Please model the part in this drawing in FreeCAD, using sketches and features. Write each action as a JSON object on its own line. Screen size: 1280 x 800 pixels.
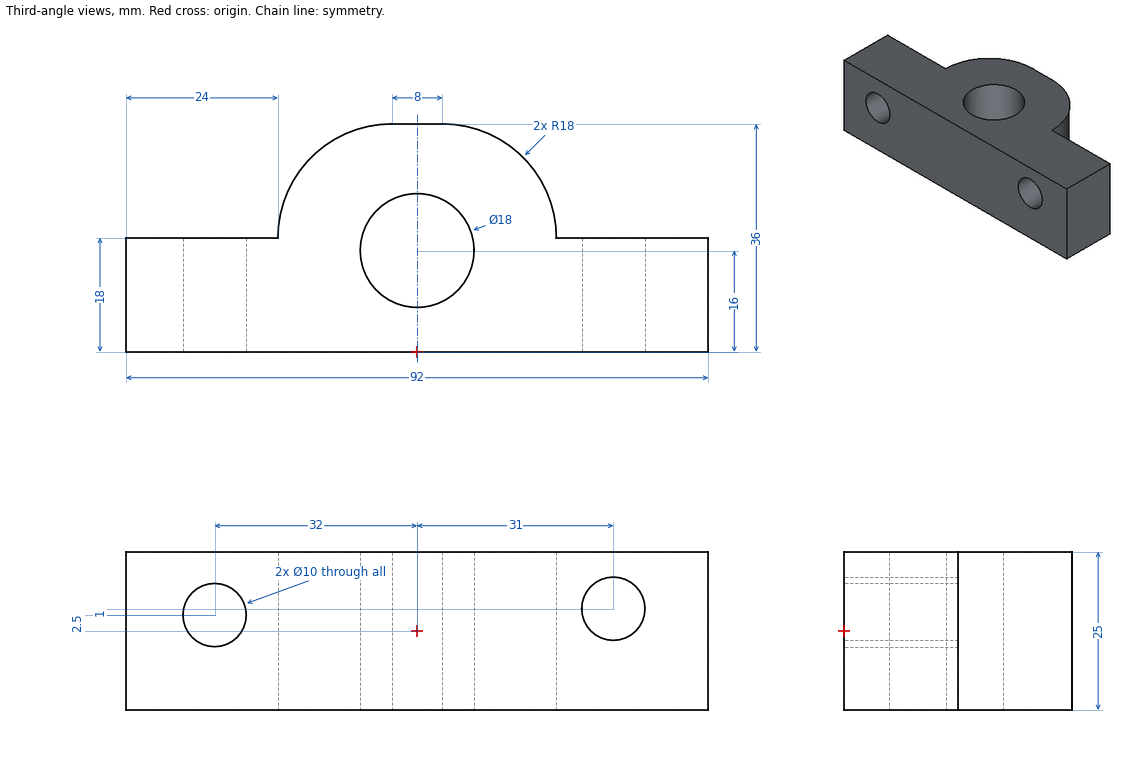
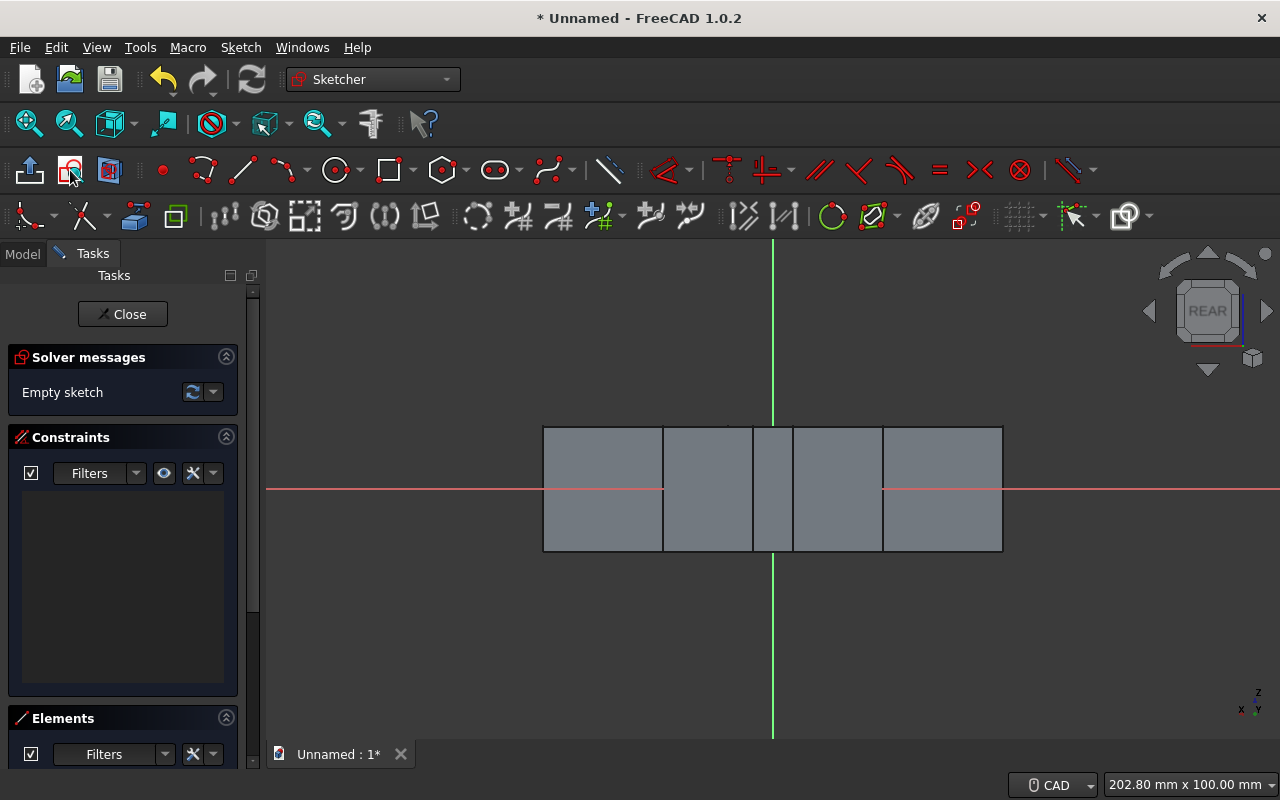
{"action": "key", "text": "q s"}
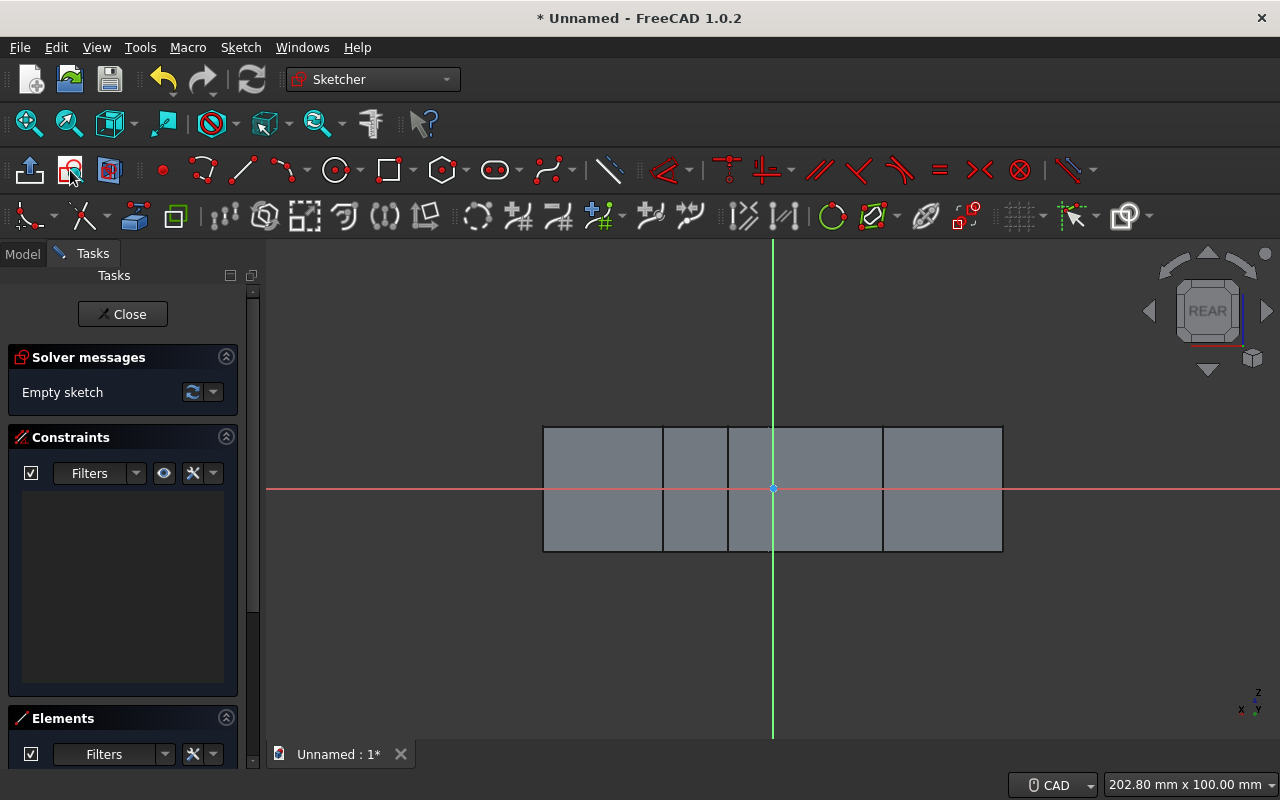
{"action": "scroll", "coordinate": [920, 444], "scroll_direction": "up", "scroll_amount": 2}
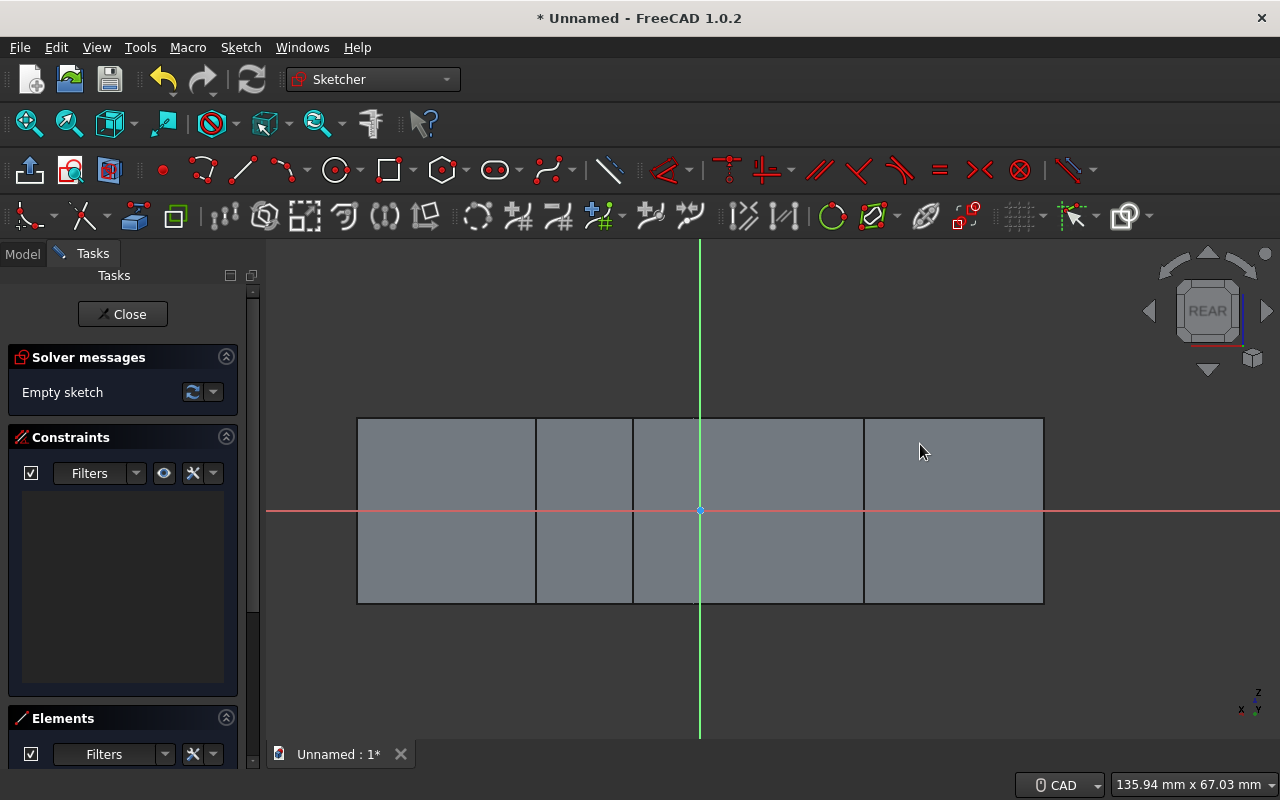
{"action": "left_click", "coordinate": [336, 170]}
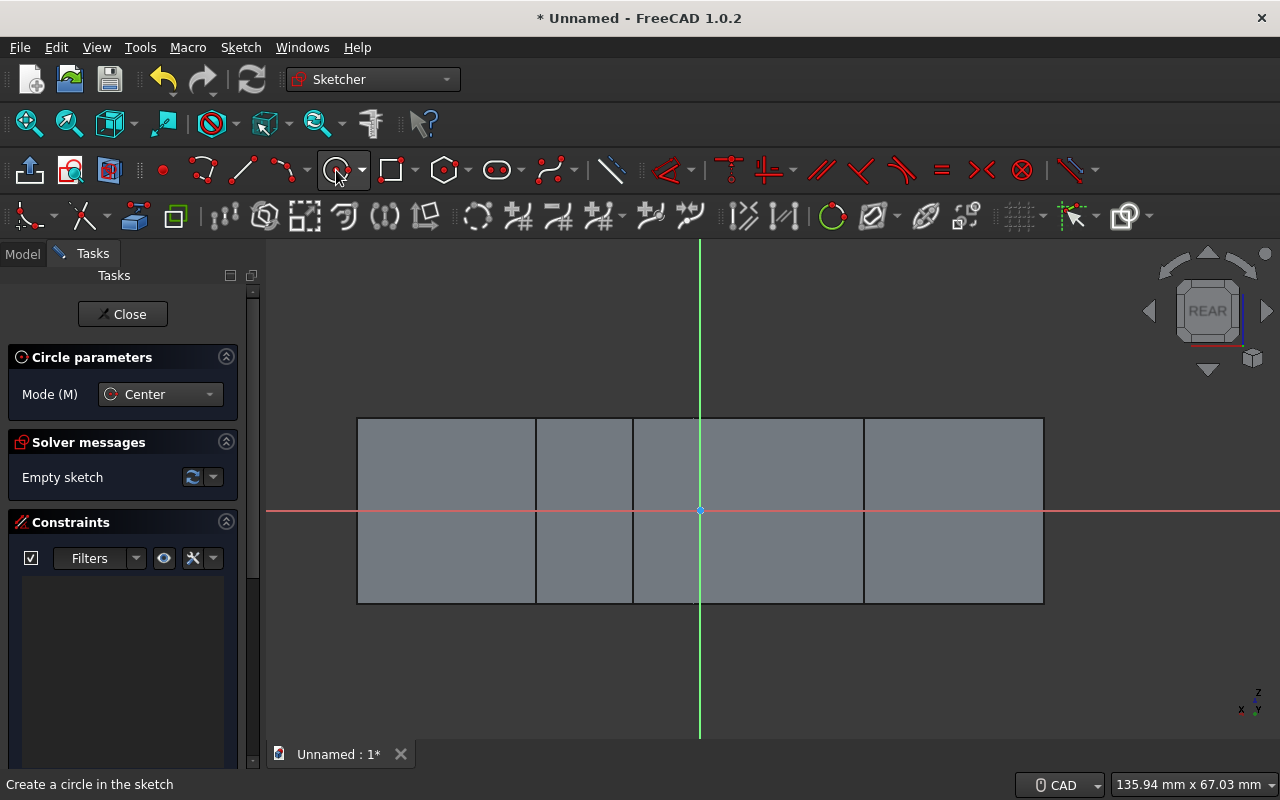
{"action": "left_click", "coordinate": [939, 492]}
{"action": "mouse_move", "coordinate": [965, 466]}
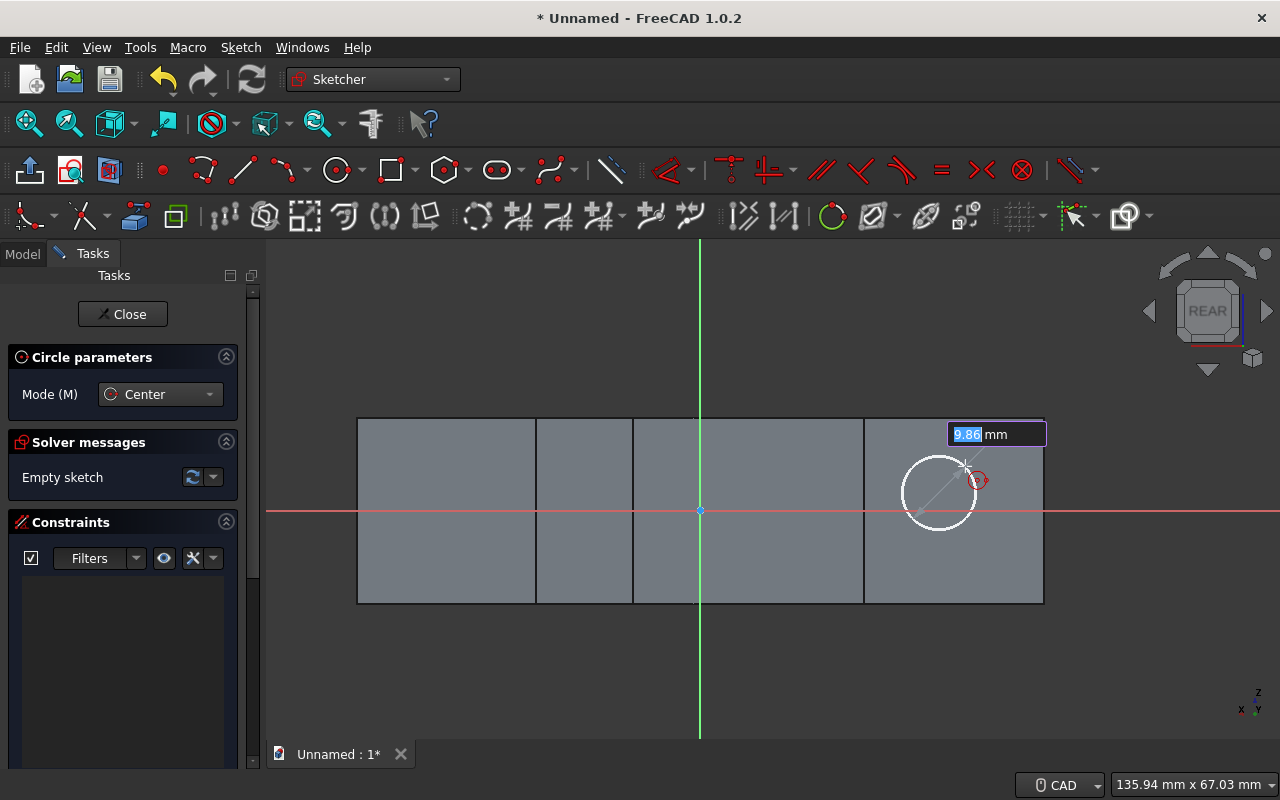
{"action": "type", "text": "10"}
{"action": "key", "text": "Return"}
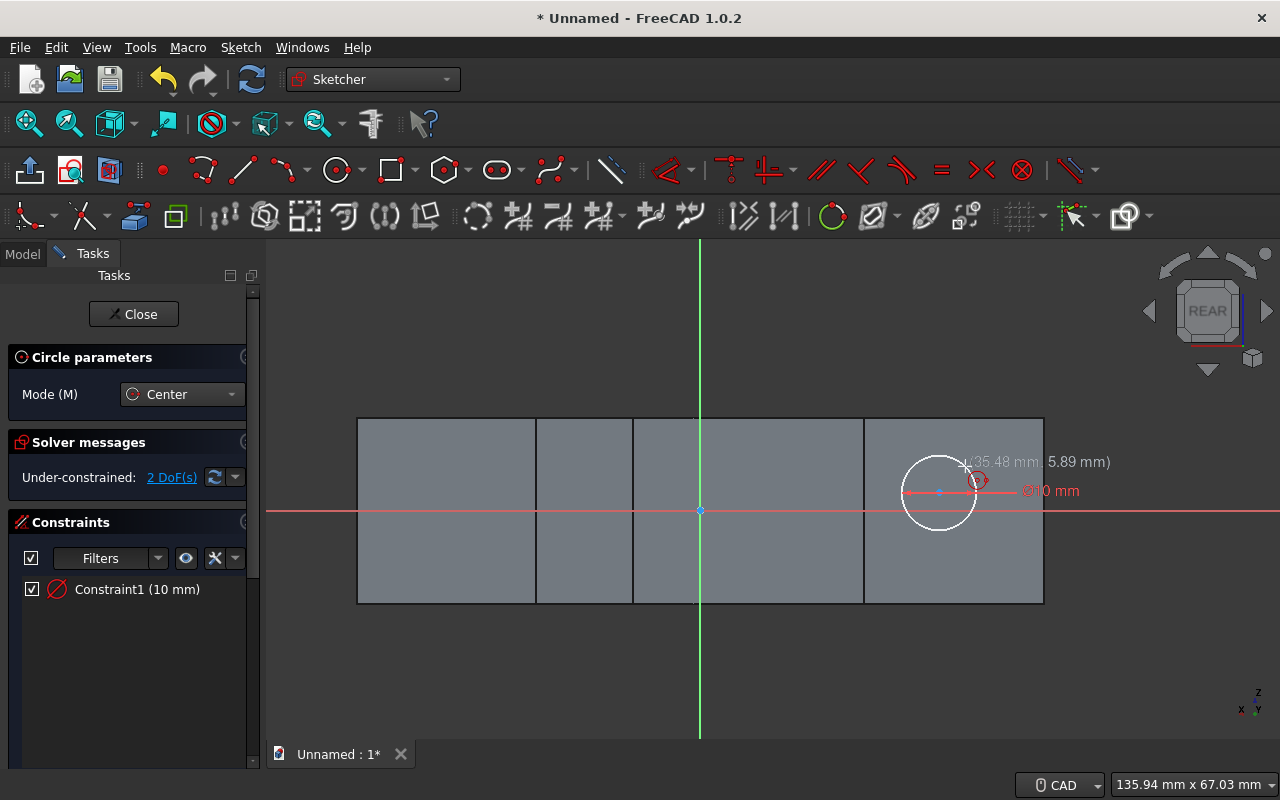
{"action": "left_click", "coordinate": [469, 485]}
{"action": "mouse_move", "coordinate": [496, 458]}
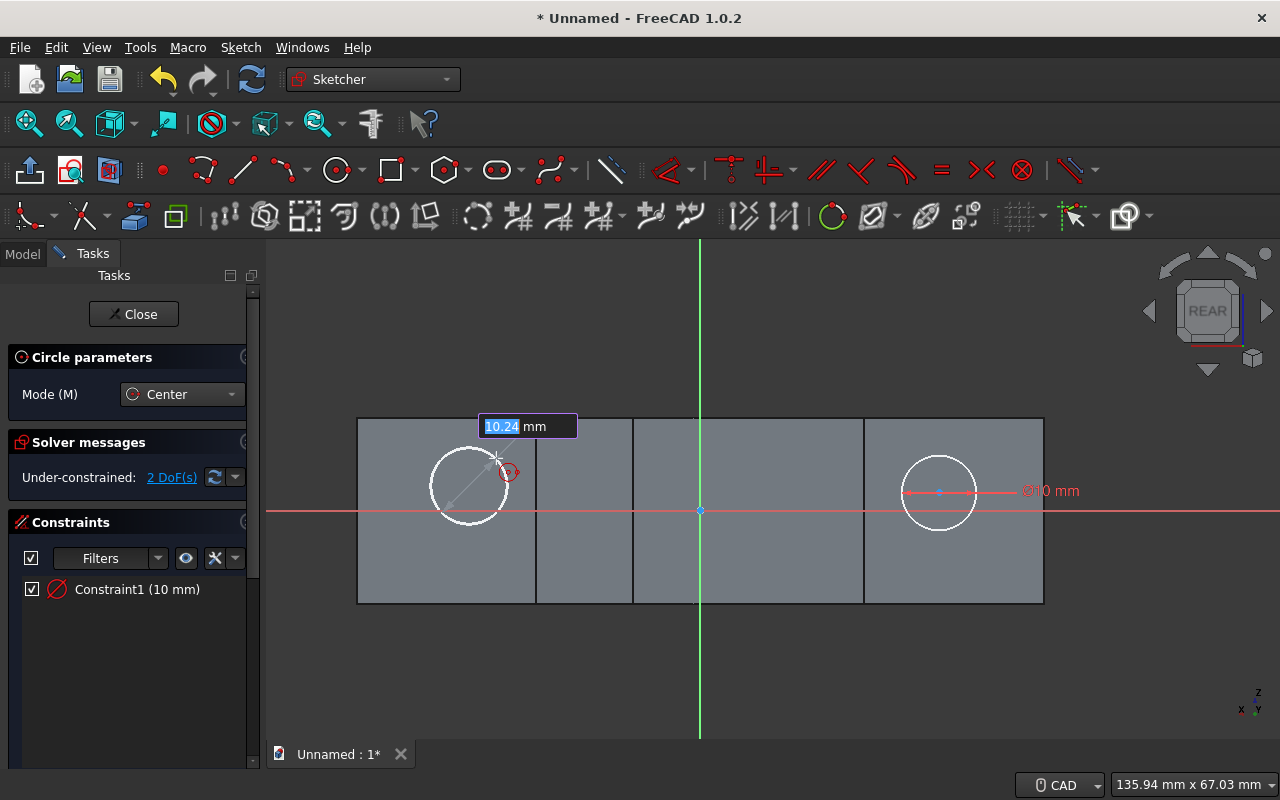
{"action": "type", "text": "10"}
{"action": "key", "text": "Return"}
{"action": "key", "text": "Escape"}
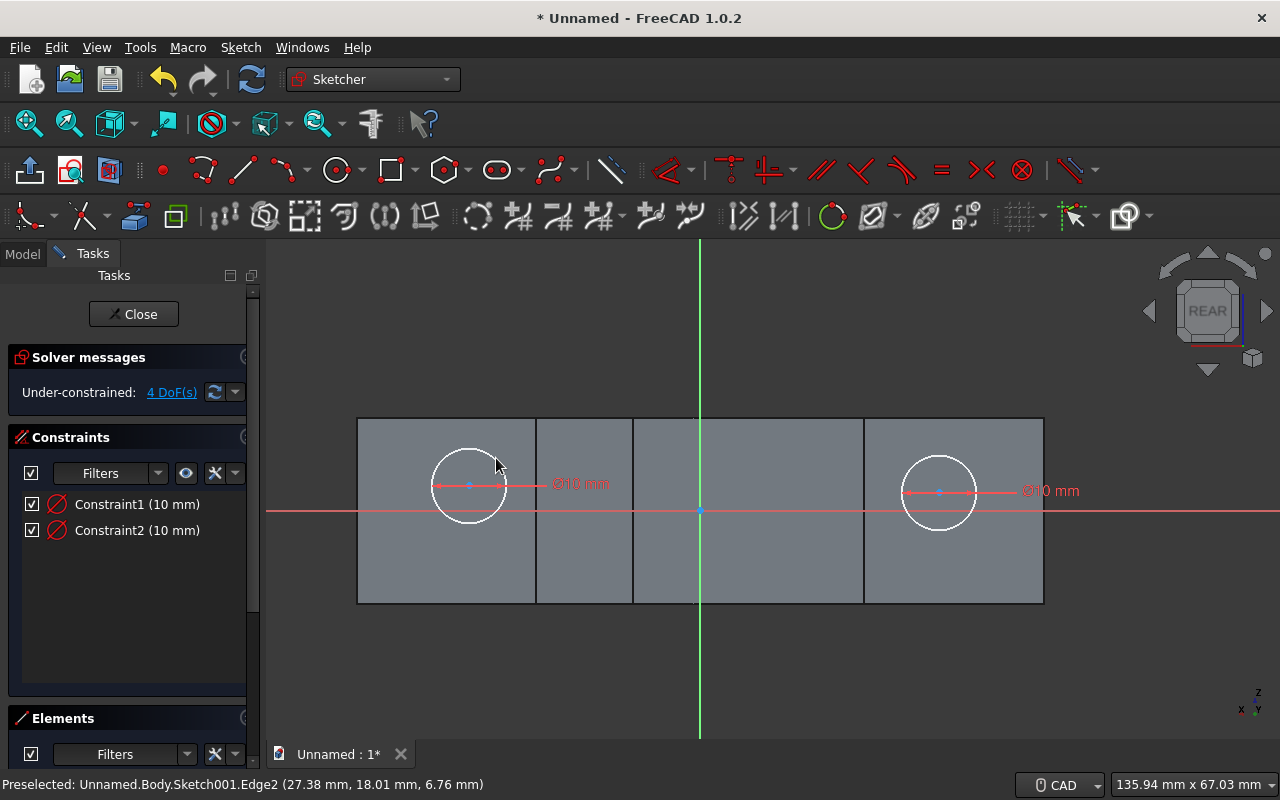
{"action": "key", "text": "d"}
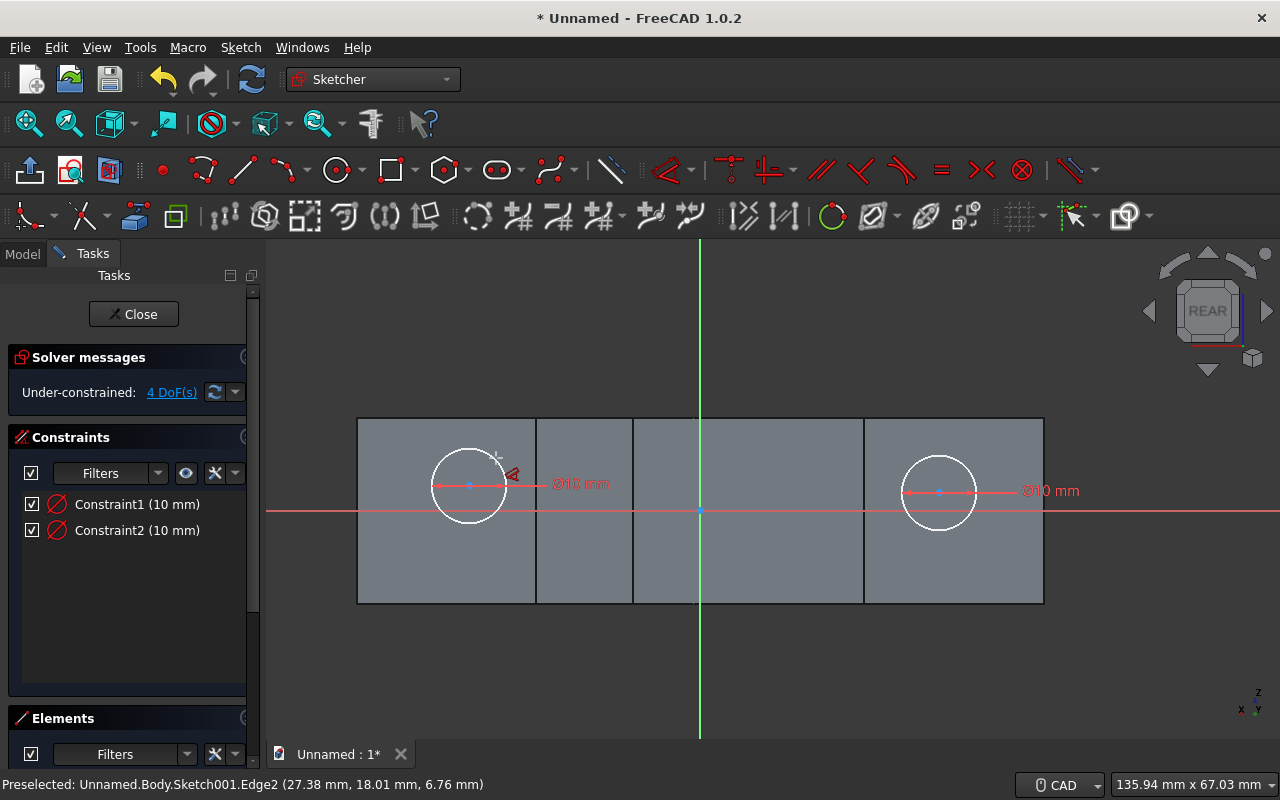
{"action": "left_click", "coordinate": [939, 493]}
{"action": "left_click", "coordinate": [820, 545]}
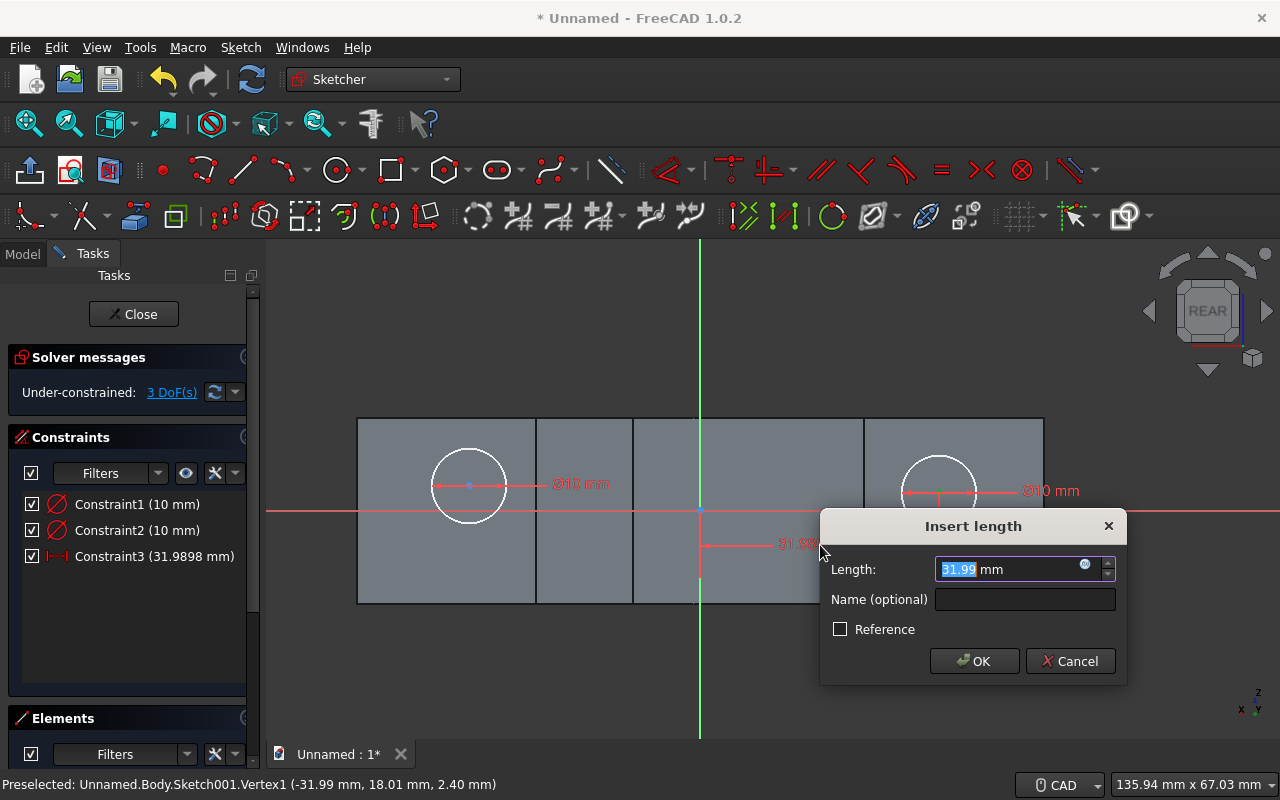
{"action": "type", "text": "32"}
{"action": "key", "text": "Return"}